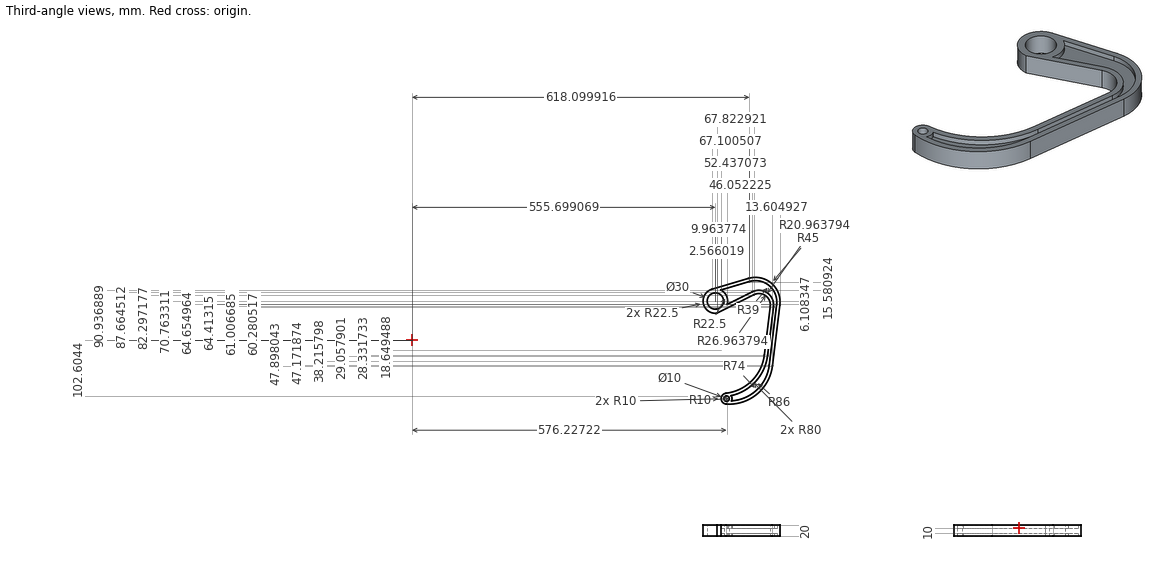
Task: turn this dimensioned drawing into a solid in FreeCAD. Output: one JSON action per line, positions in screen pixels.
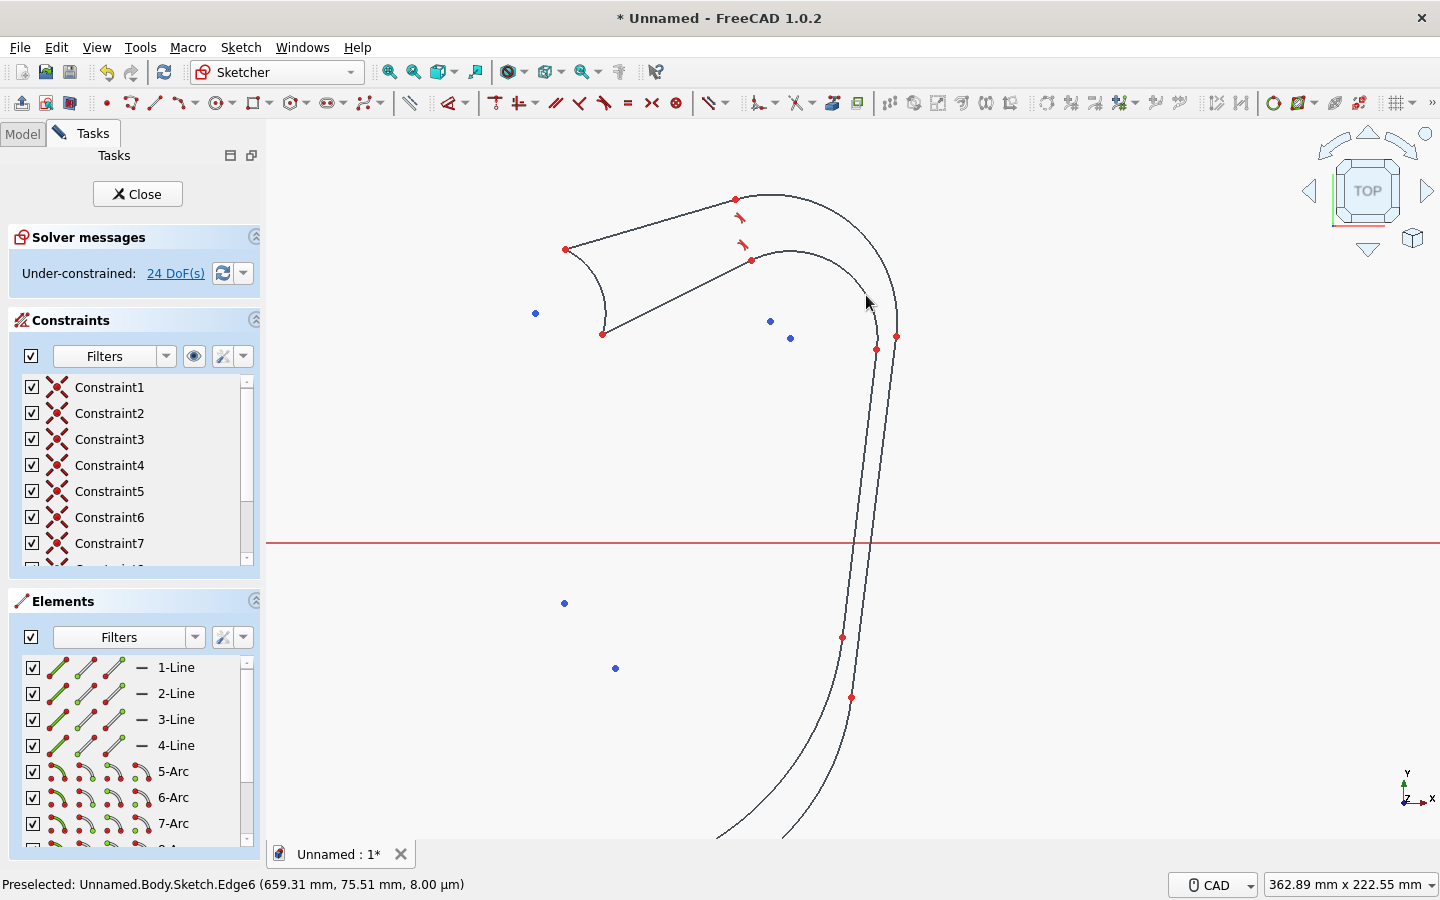
{"action": "left_click", "coordinate": [867, 436]}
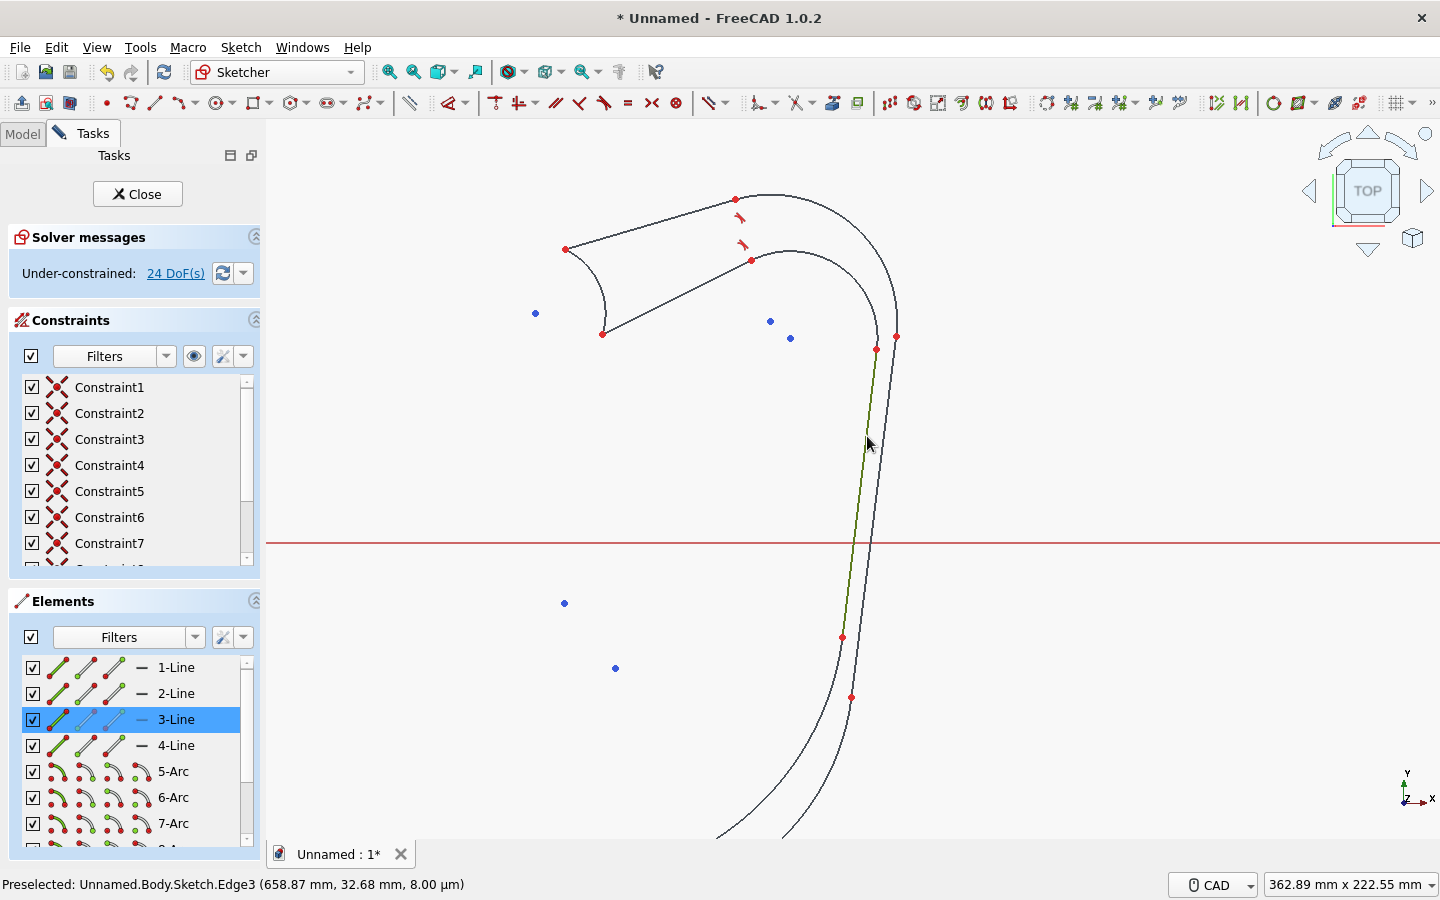
{"action": "left_click", "coordinate": [866, 295]}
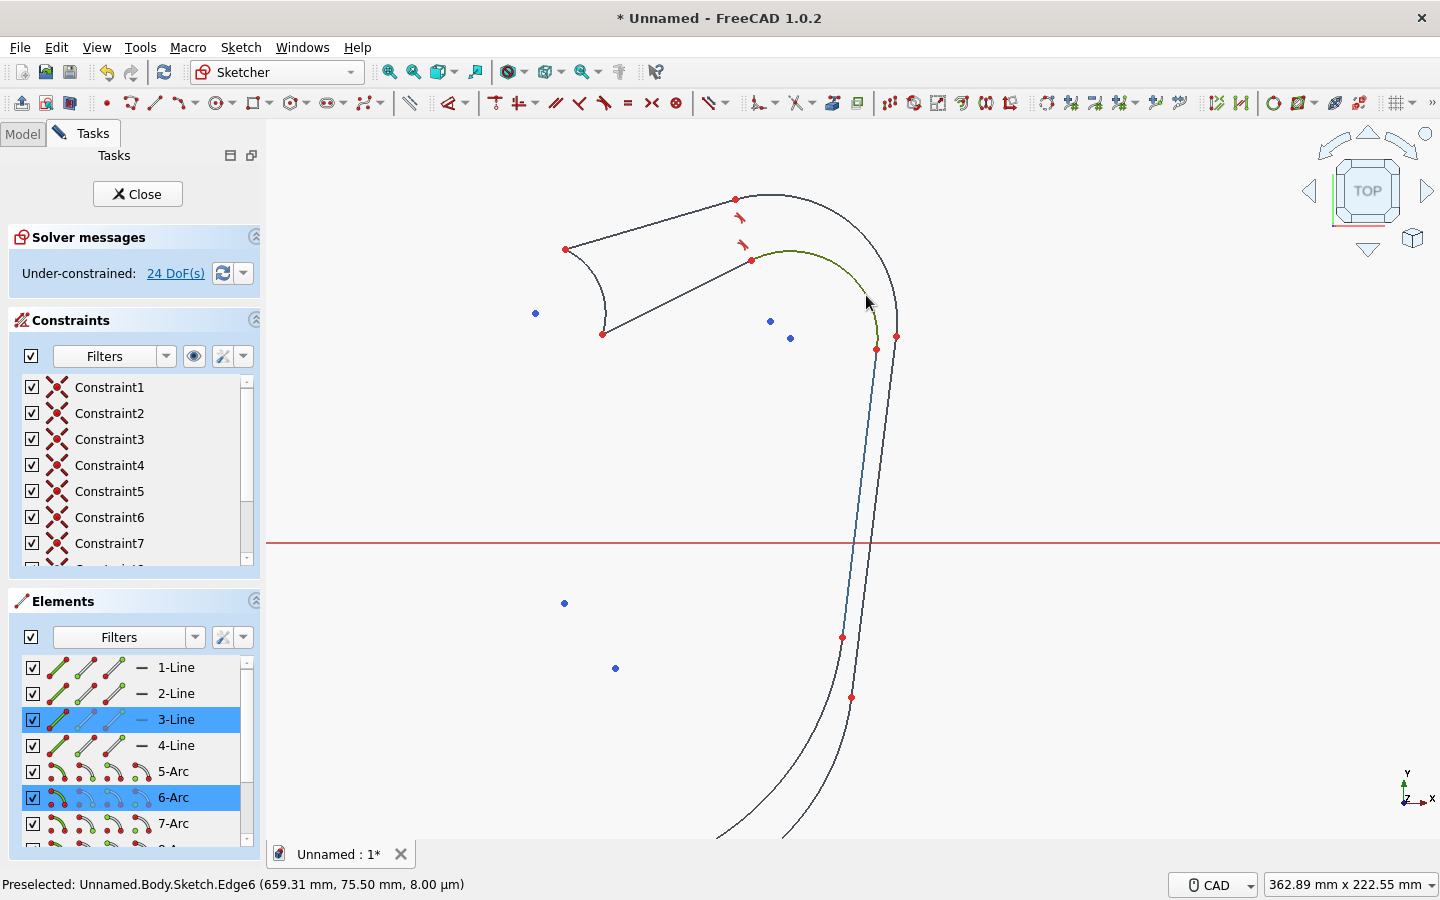
{"action": "left_click", "coordinate": [604, 104]}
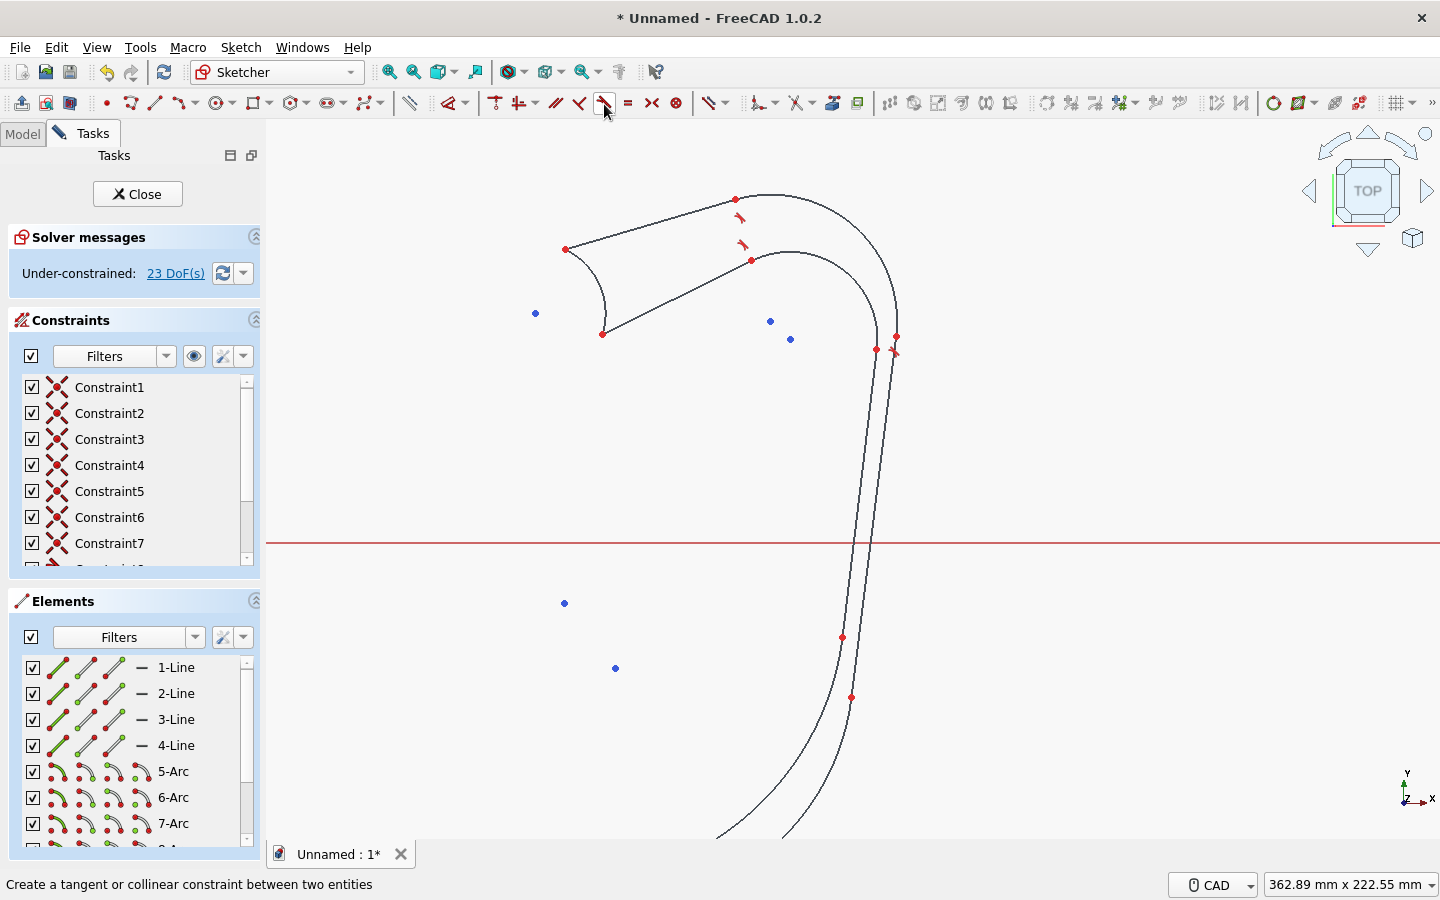
{"action": "left_click", "coordinate": [865, 589]}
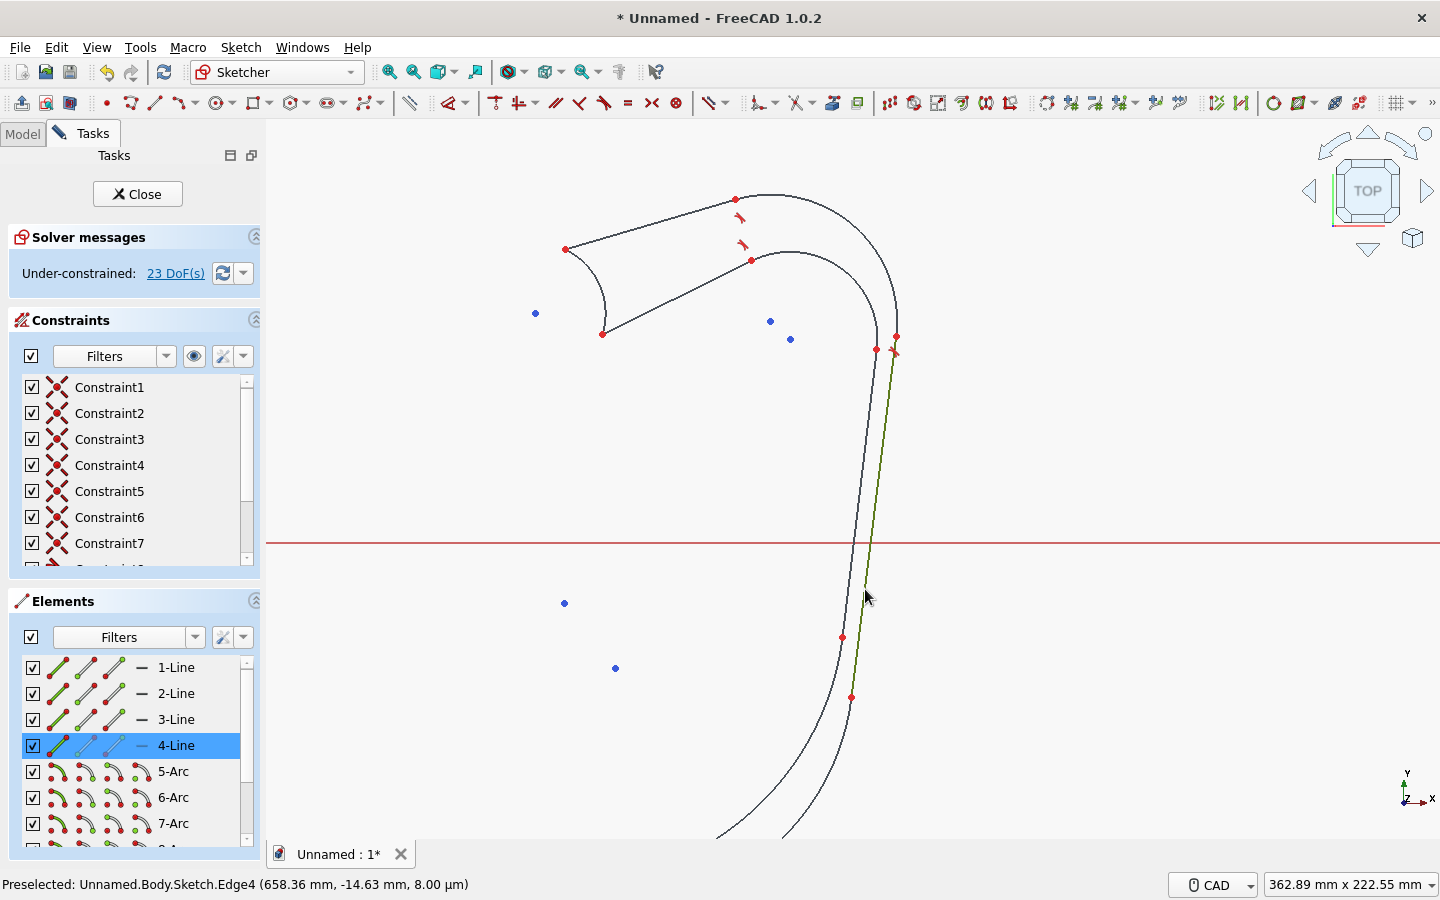
{"action": "left_click", "coordinate": [883, 263]}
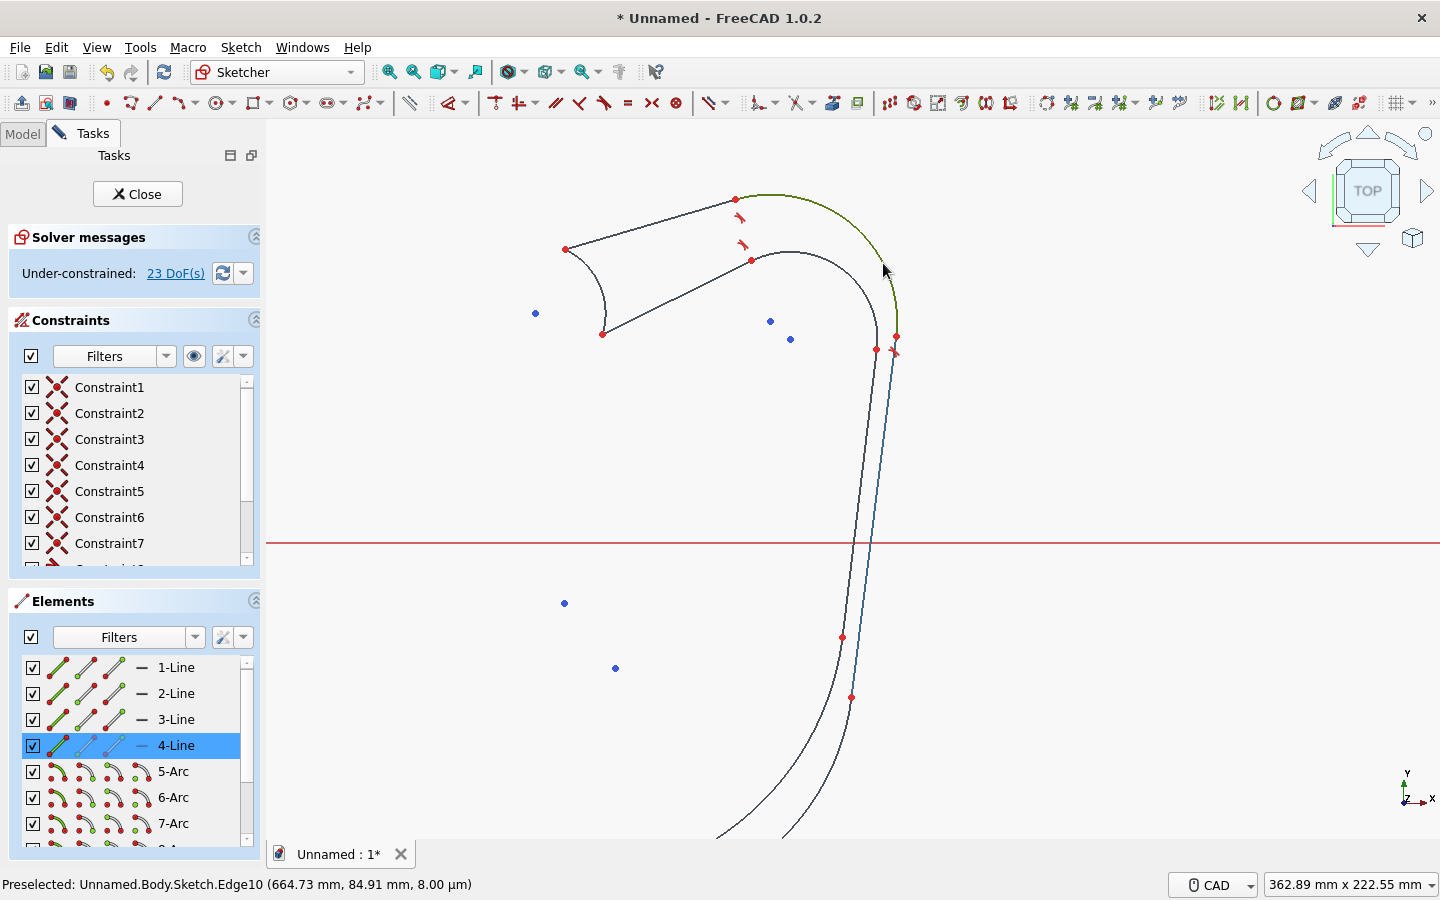
{"action": "left_click", "coordinate": [604, 104]}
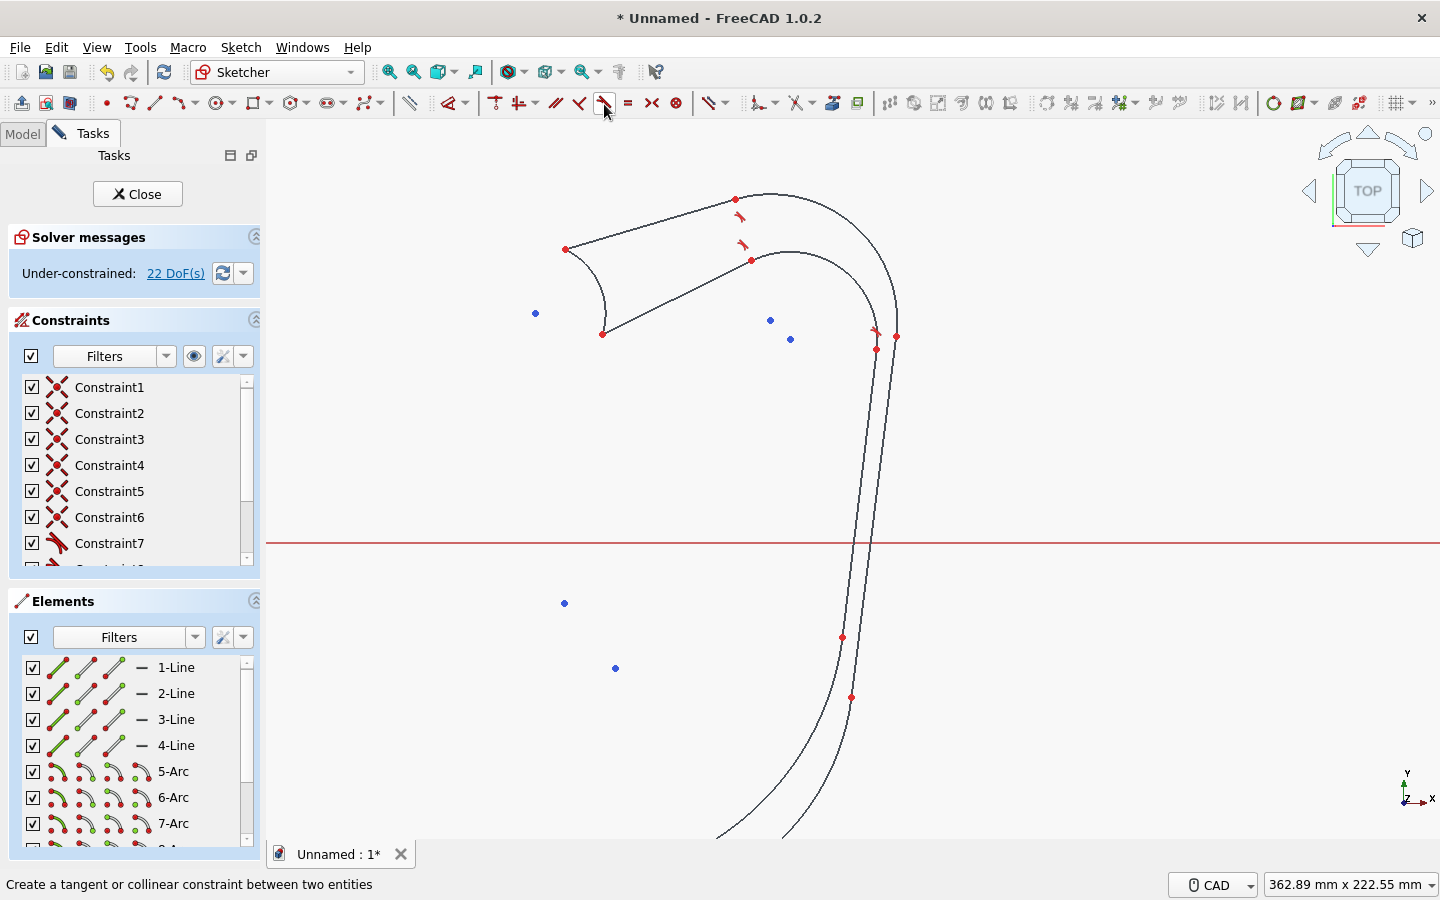
{"action": "left_click", "coordinate": [448, 104]}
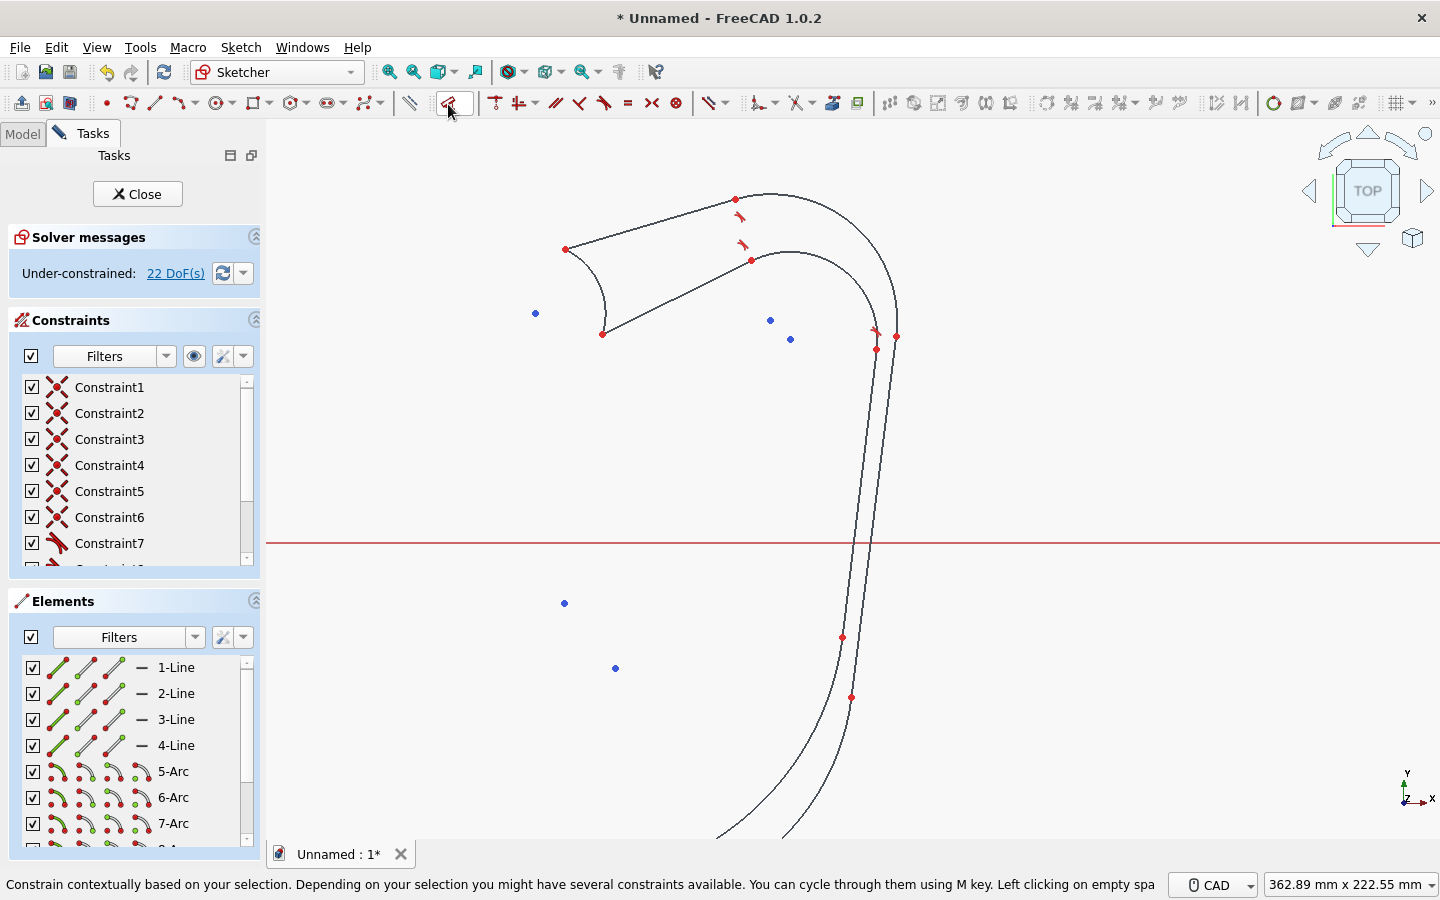
{"action": "left_click", "coordinate": [605, 305]}
{"action": "left_click", "coordinate": [637, 301]}